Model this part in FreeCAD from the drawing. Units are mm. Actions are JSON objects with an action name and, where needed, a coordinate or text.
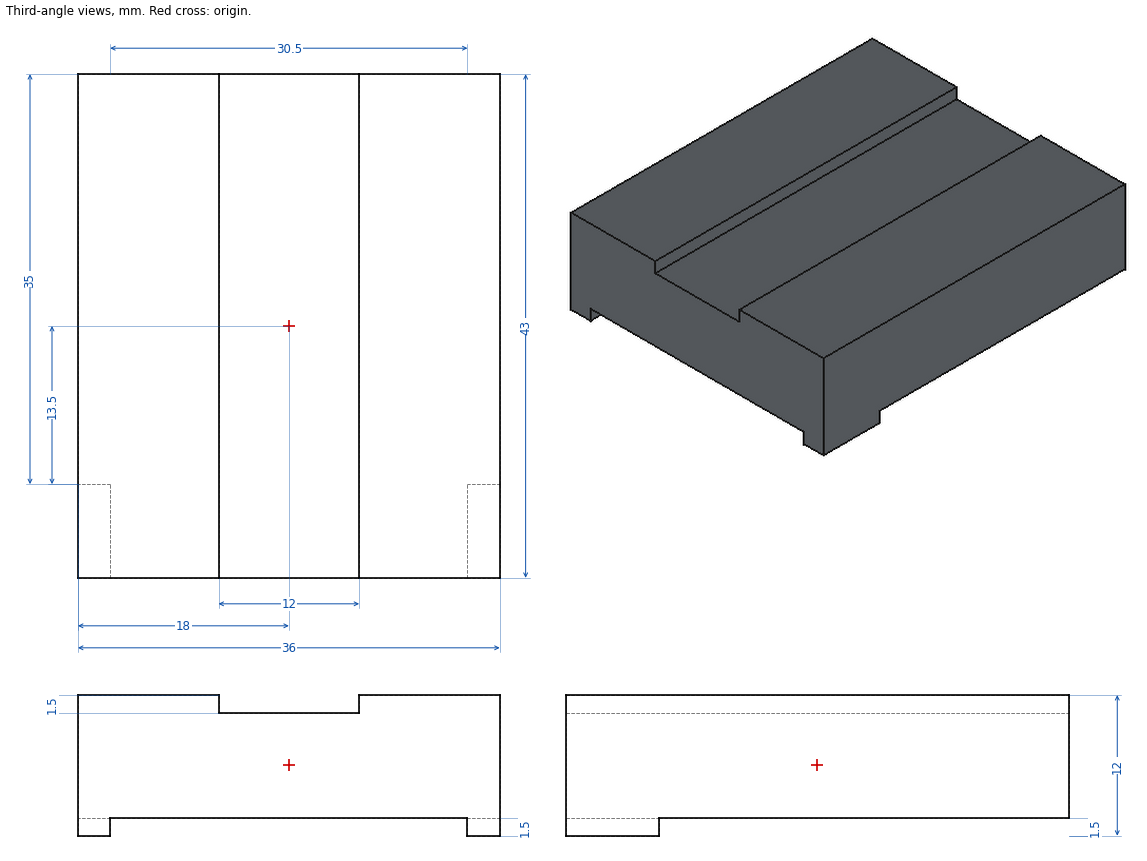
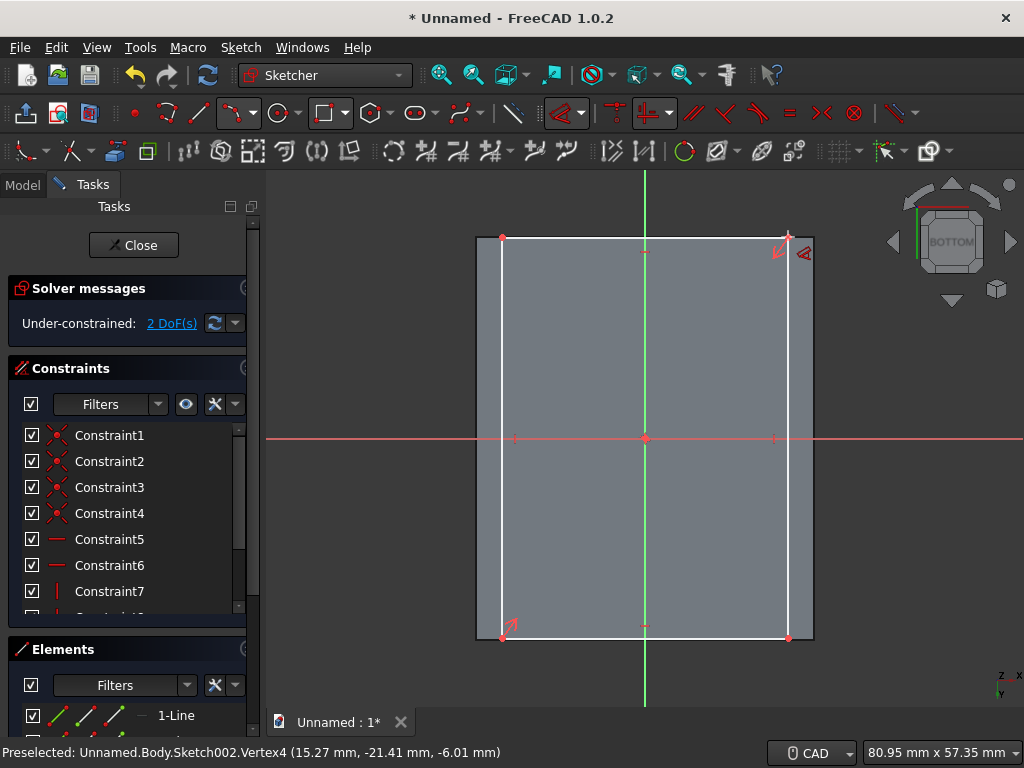
{"action": "left_click", "coordinate": [788, 519]}
{"action": "left_click", "coordinate": [822, 346]}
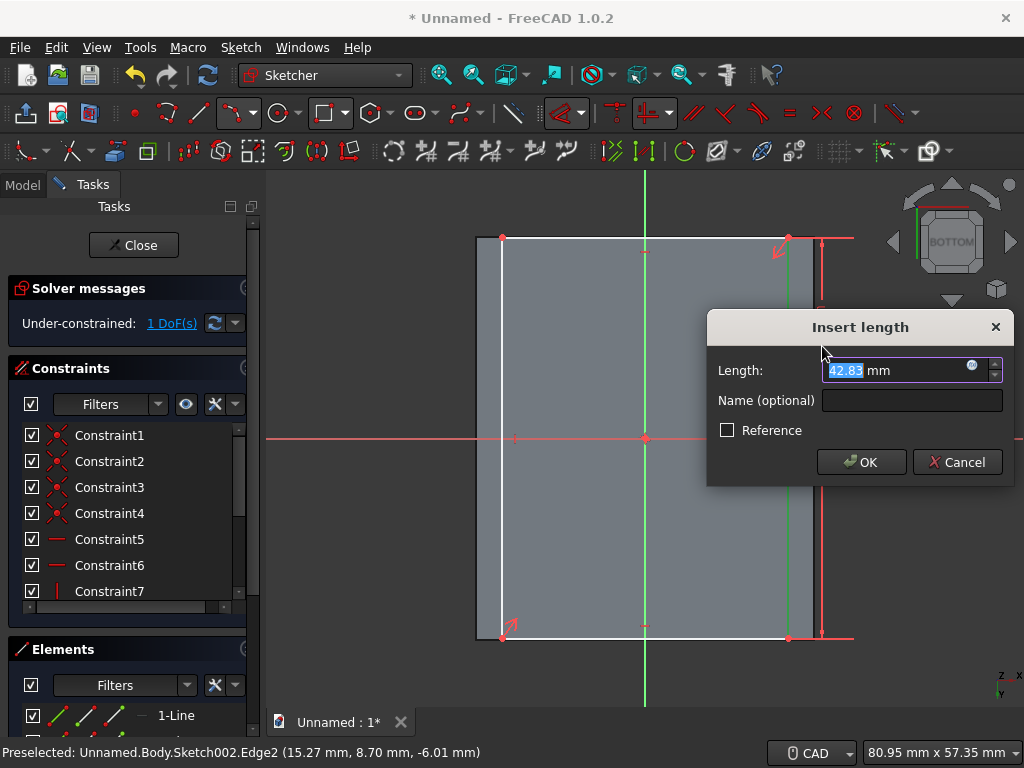
{"action": "type", "text": "43"}
{"action": "key", "text": "Return"}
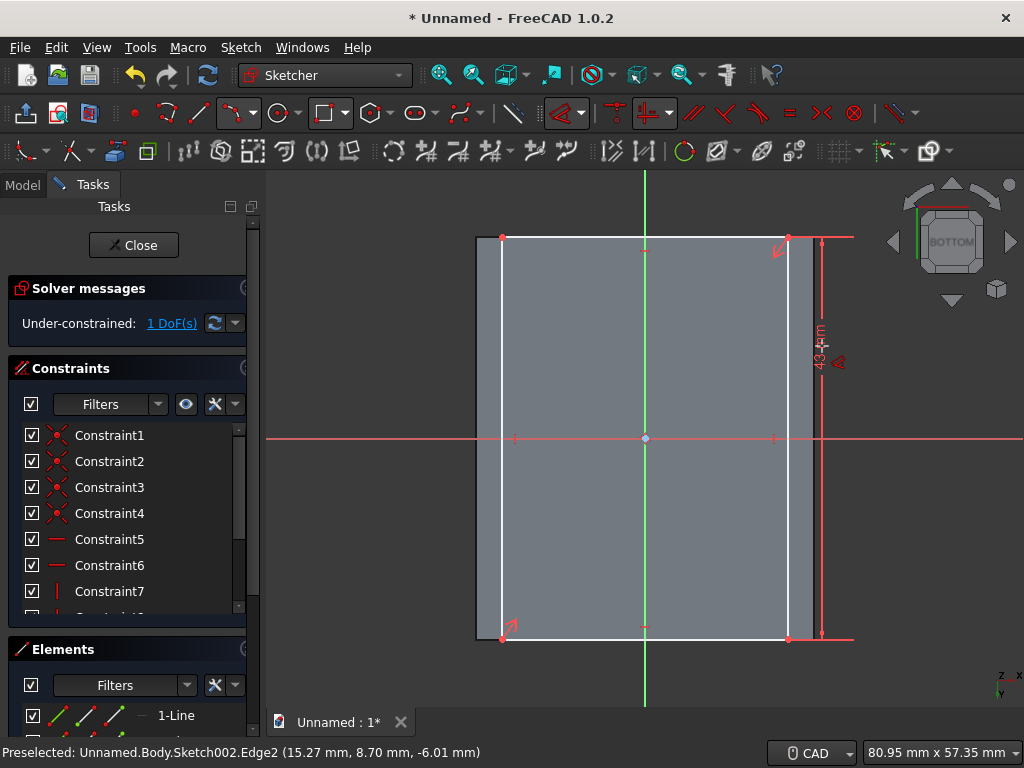
{"action": "left_click", "coordinate": [588, 640]}
{"action": "left_click", "coordinate": [579, 674]}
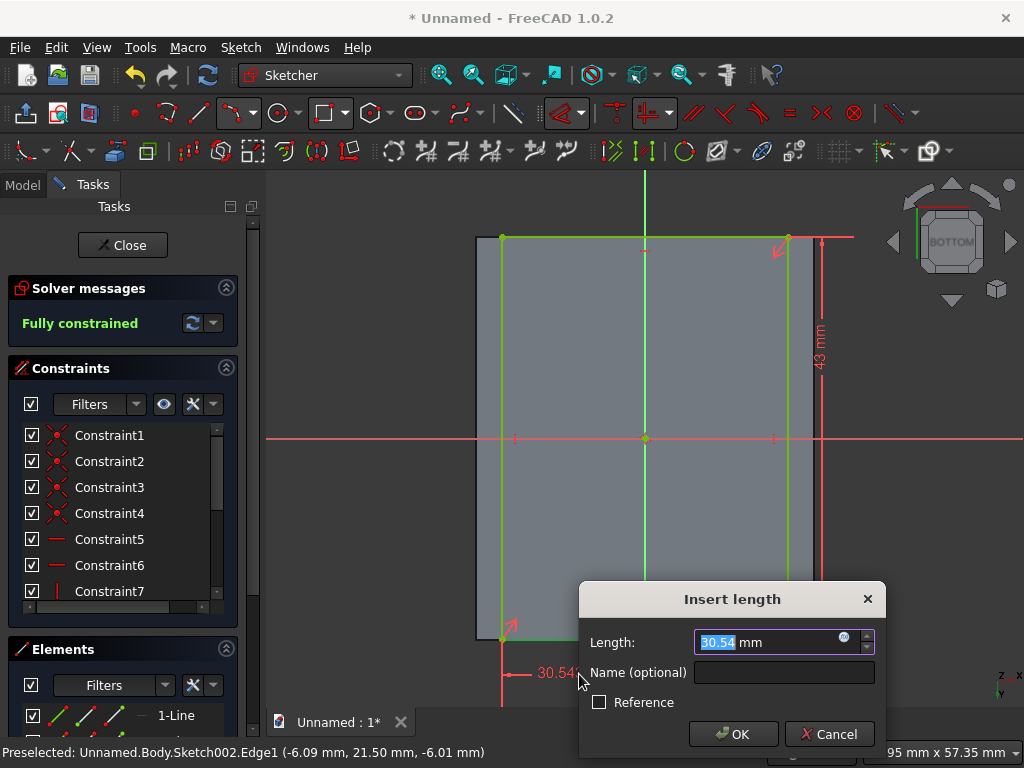
{"action": "type", "text": "30.5"}
{"action": "key", "text": "Return"}
{"action": "key", "text": "Escape"}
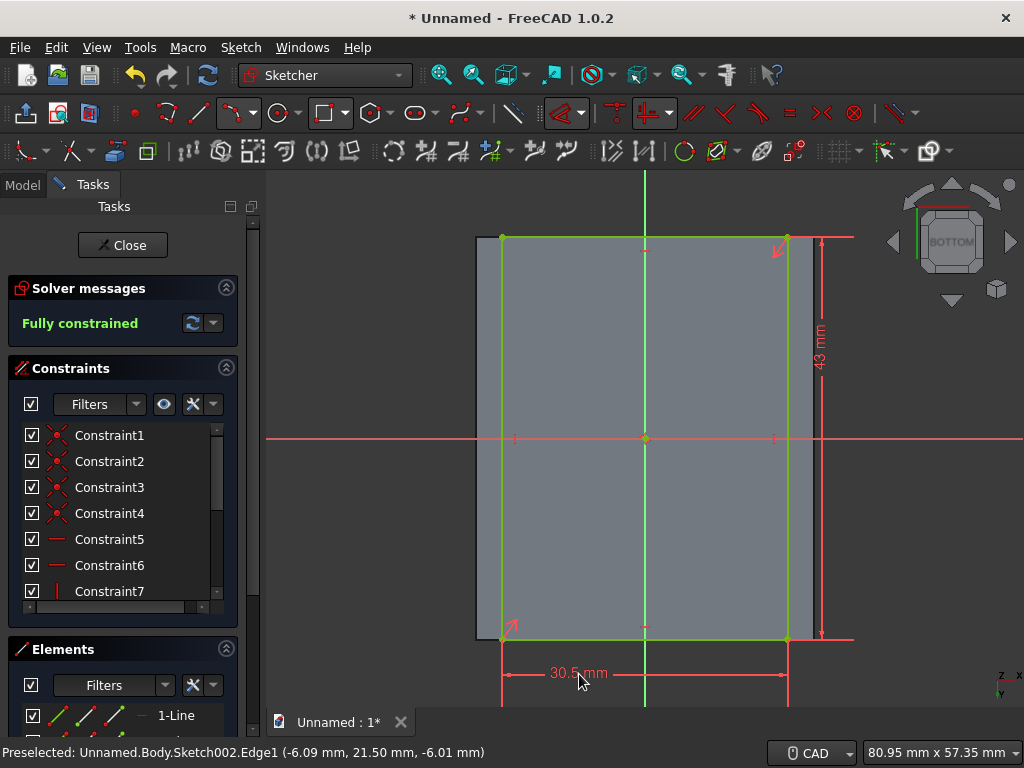
{"action": "left_click", "coordinate": [123, 245]}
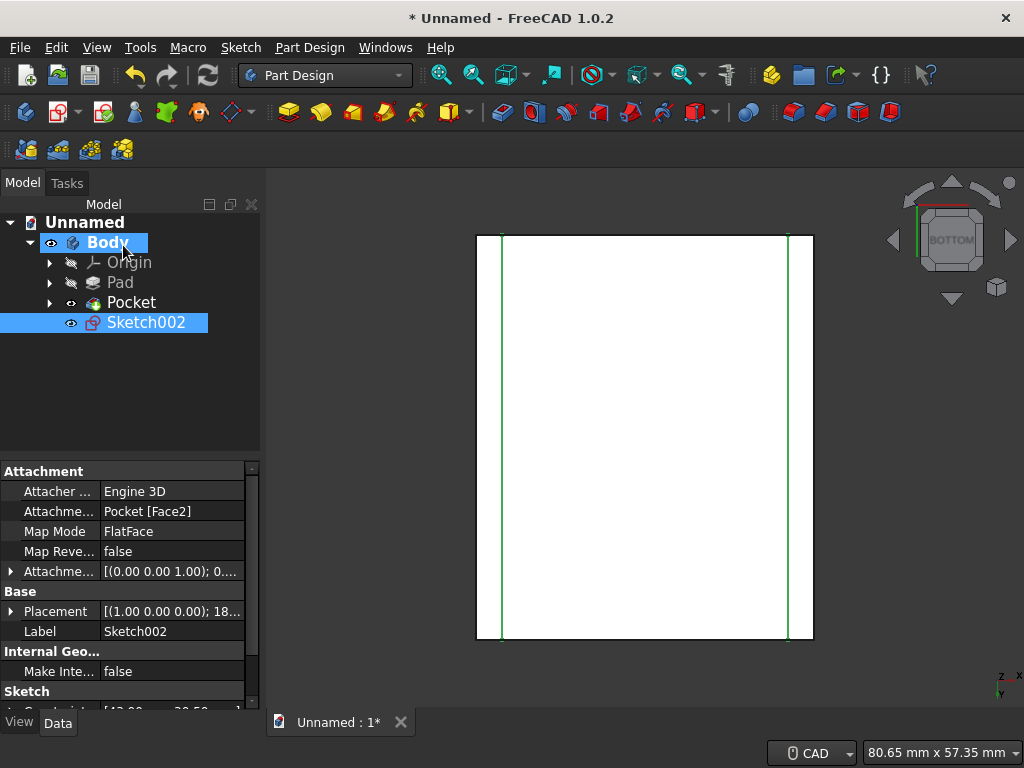
{"action": "left_click", "coordinate": [504, 112]}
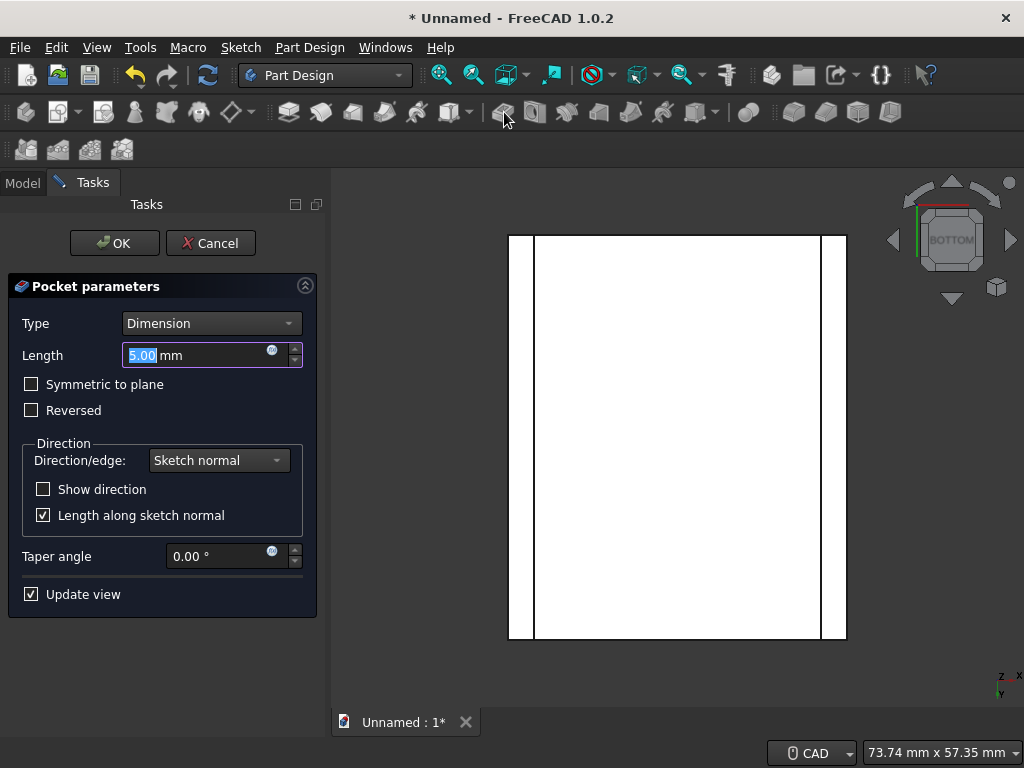
{"action": "type", "text": "1.5"}
{"action": "key", "text": "Tab"}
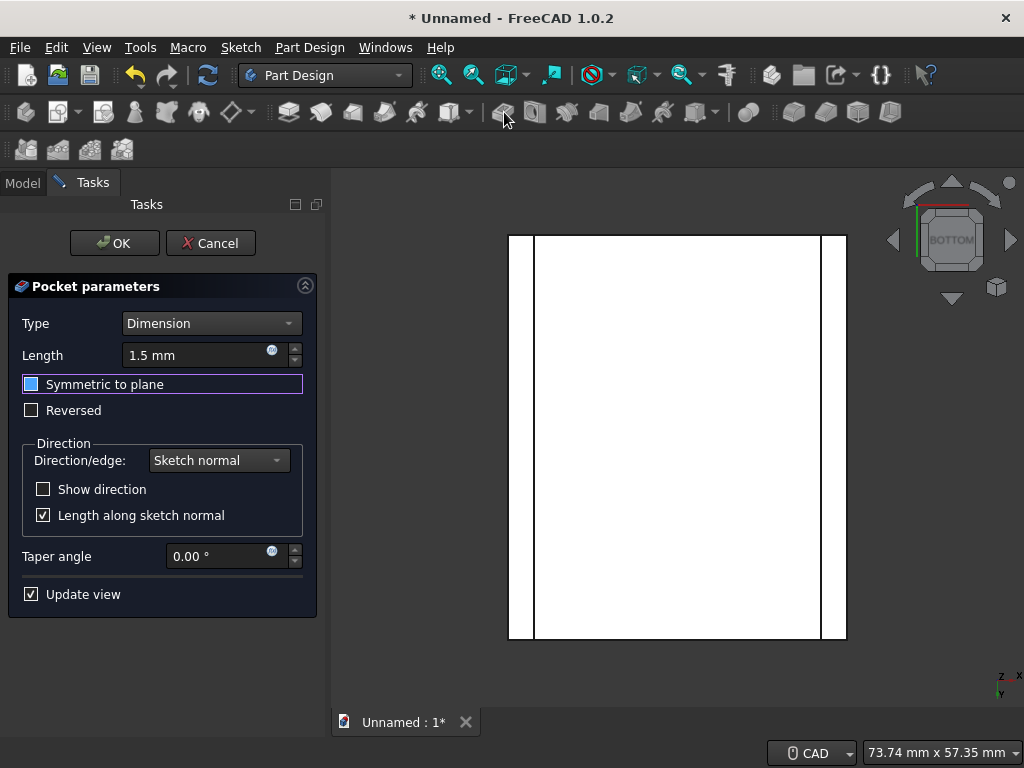
{"action": "left_click", "coordinate": [115, 243]}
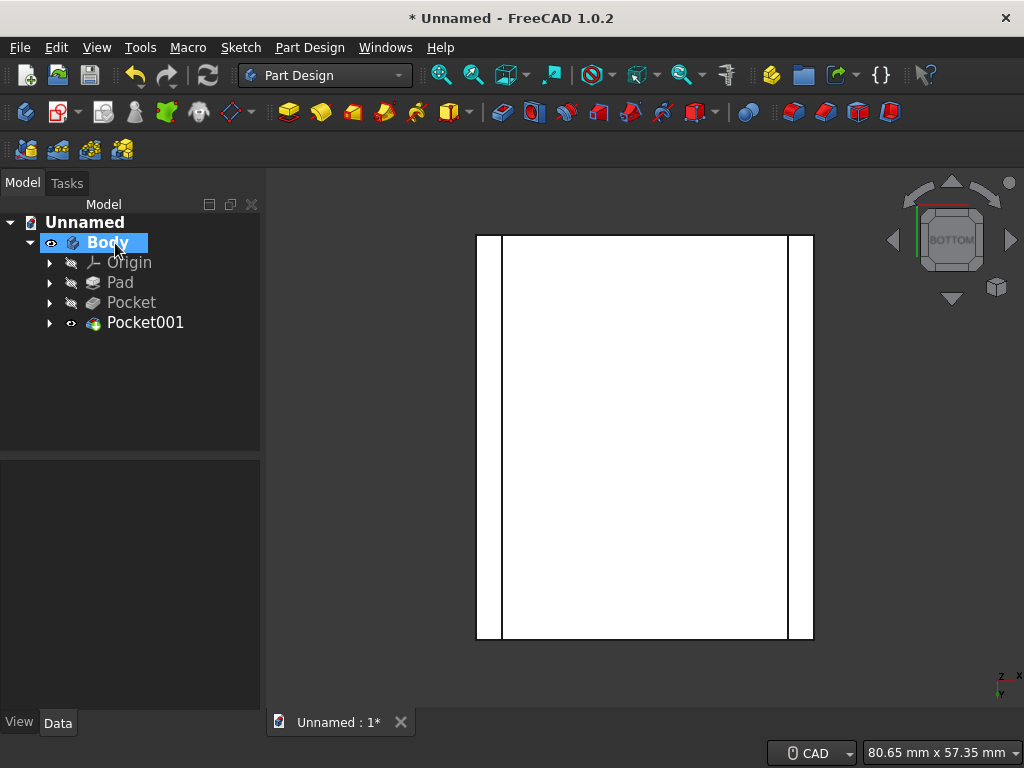
{"action": "left_click", "coordinate": [801, 610]}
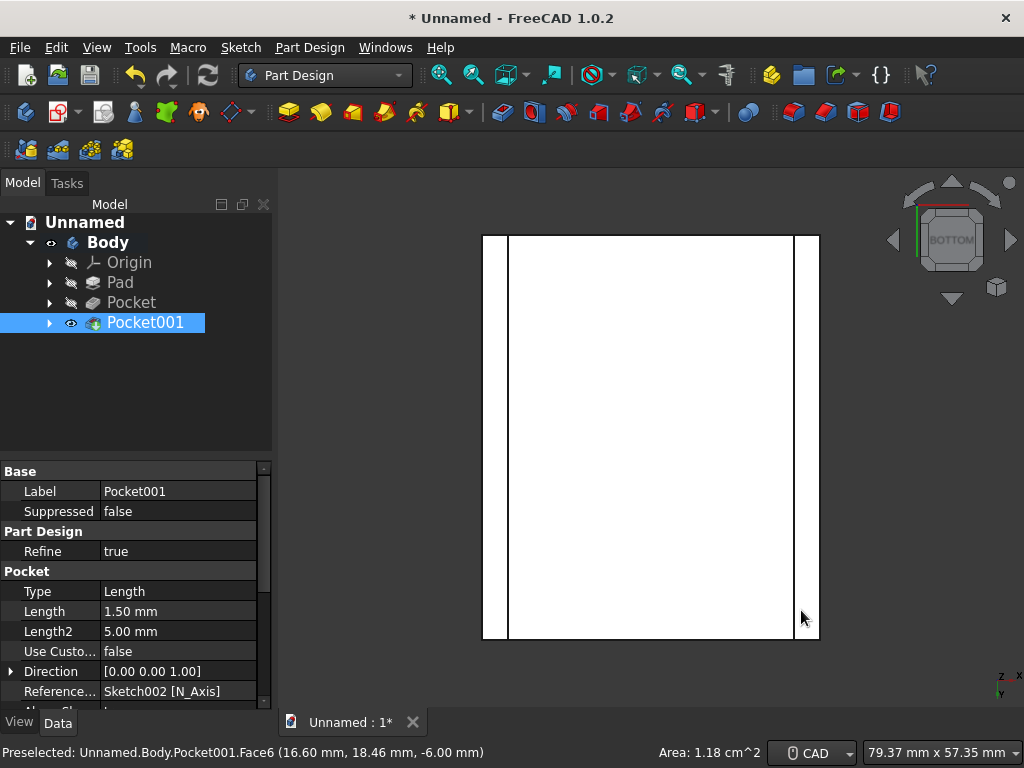
{"action": "left_click", "coordinate": [58, 112]}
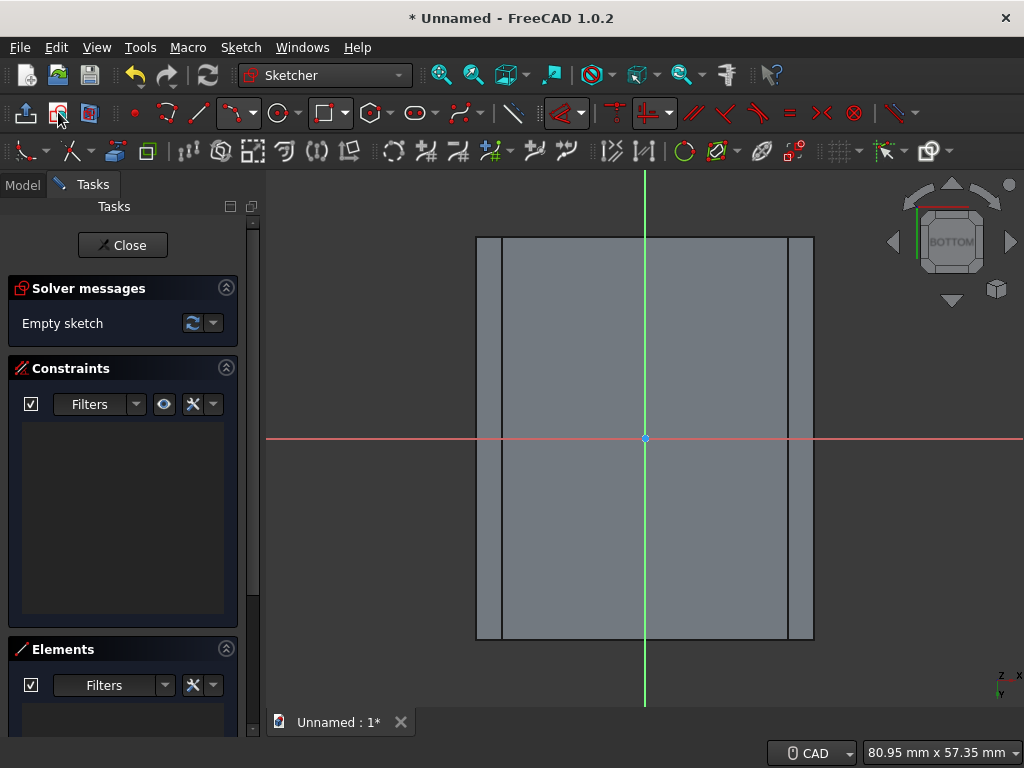
{"action": "key", "text": "g r"}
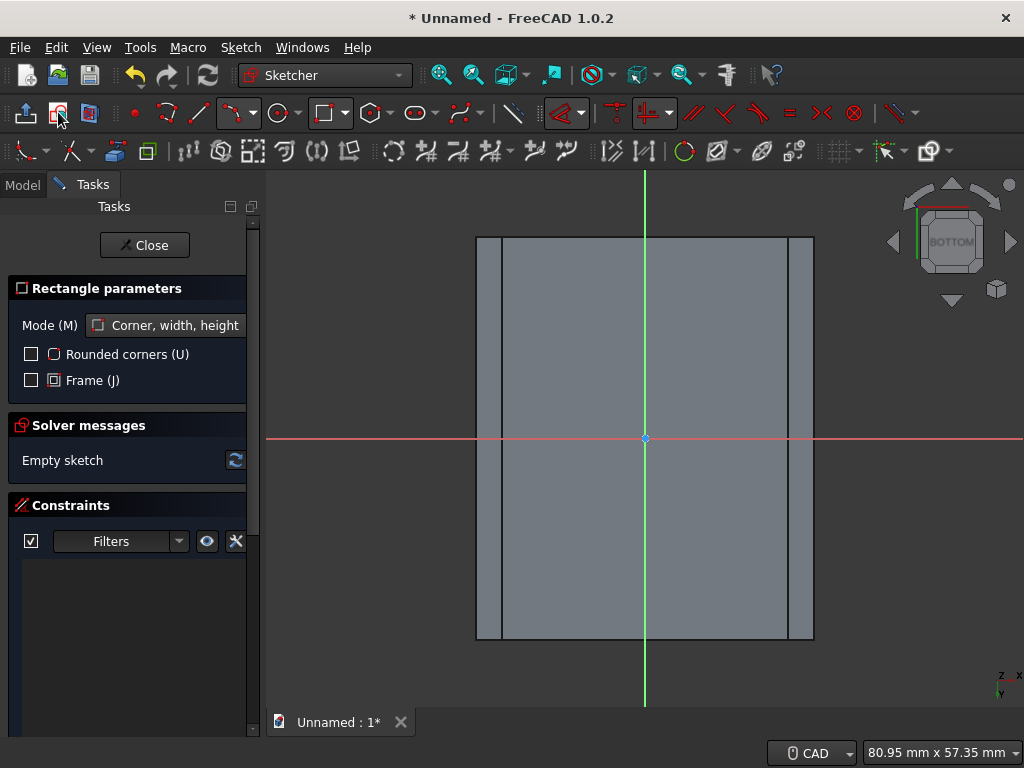
{"action": "left_click", "coordinate": [476, 312]}
{"action": "left_click", "coordinate": [814, 640]}
{"action": "key", "text": "Escape"}